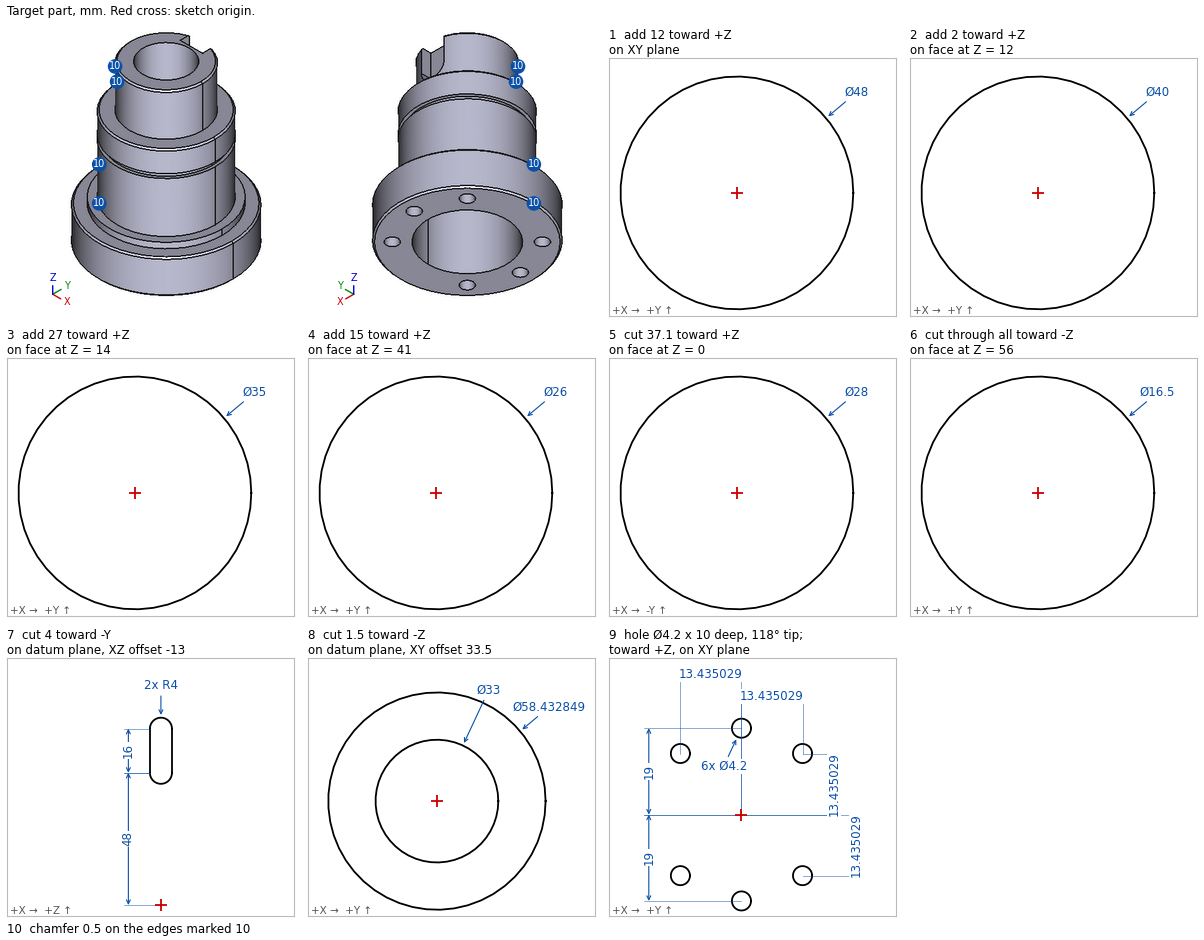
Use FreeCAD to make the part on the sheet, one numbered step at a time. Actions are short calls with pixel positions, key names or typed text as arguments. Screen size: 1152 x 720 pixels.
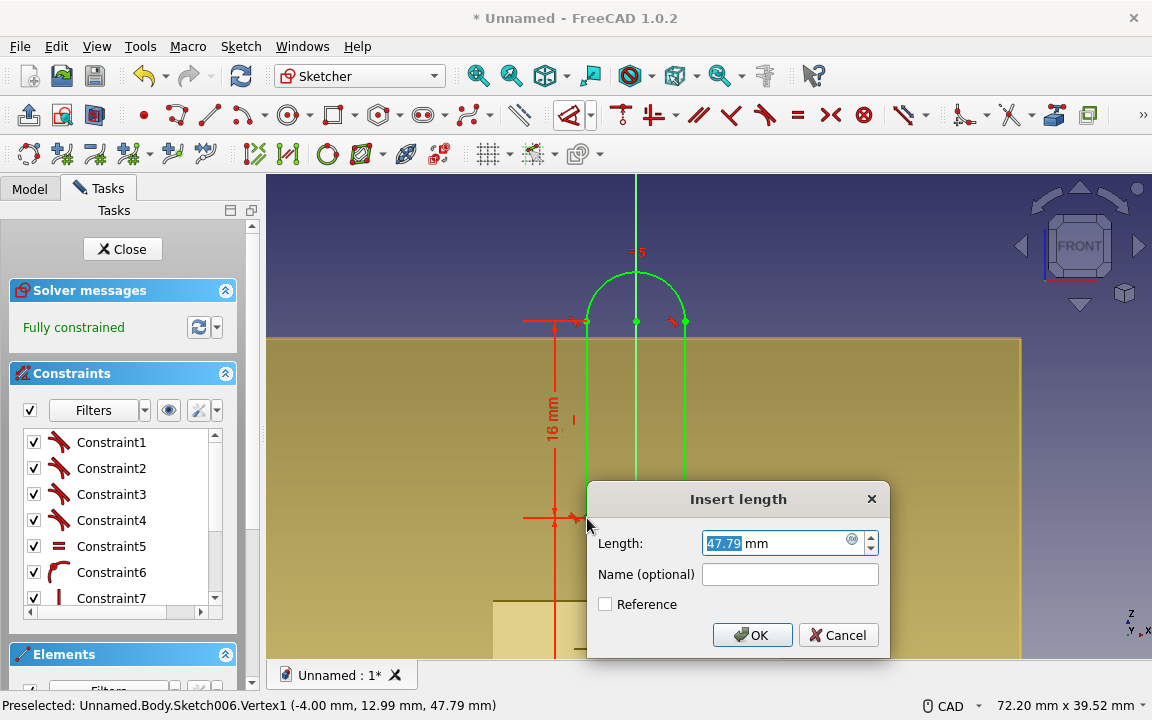
text(48)
key(Return)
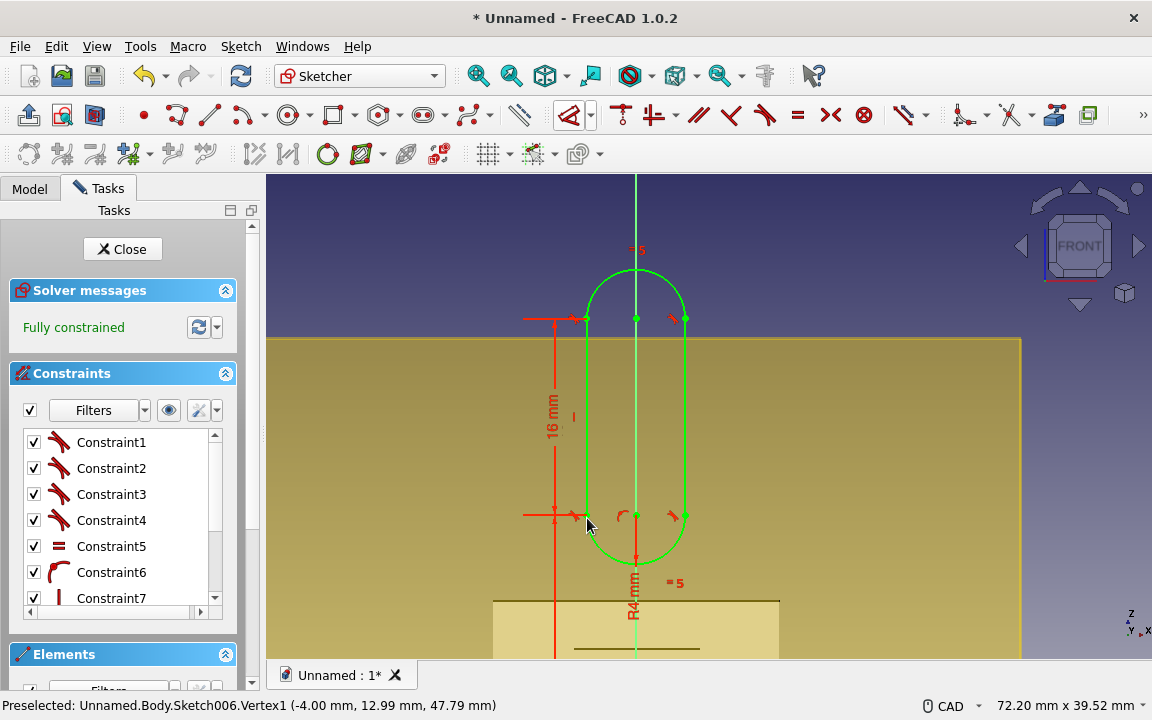
click(123, 249)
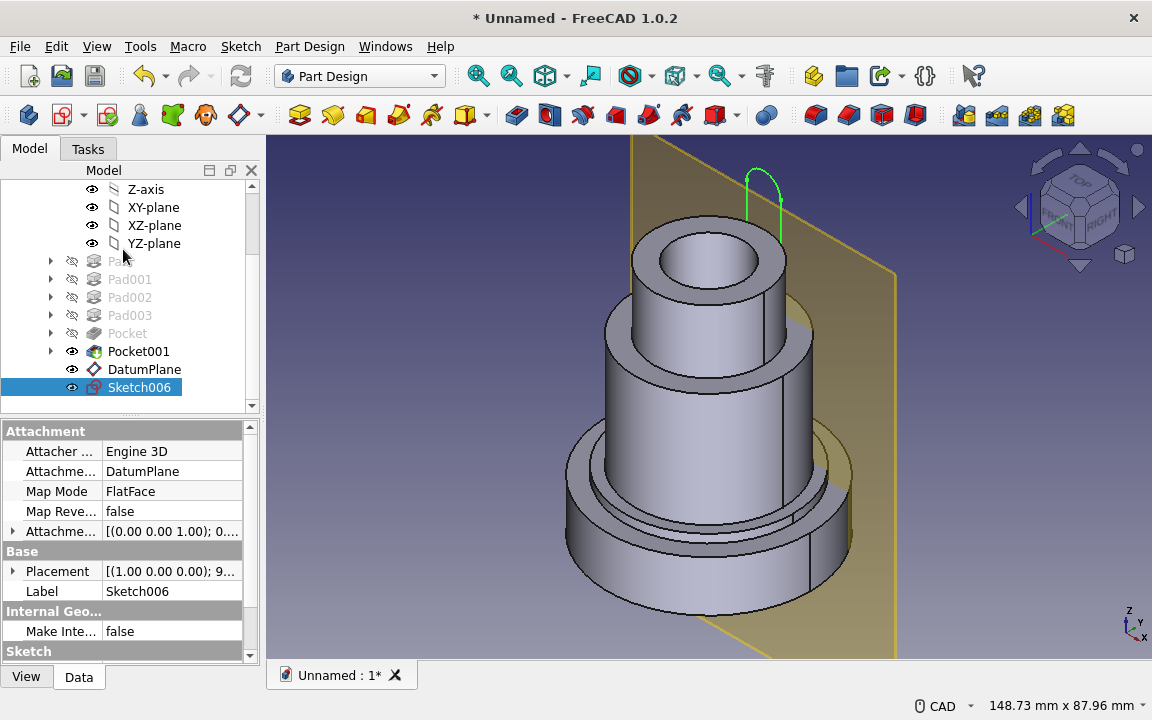
click(517, 116)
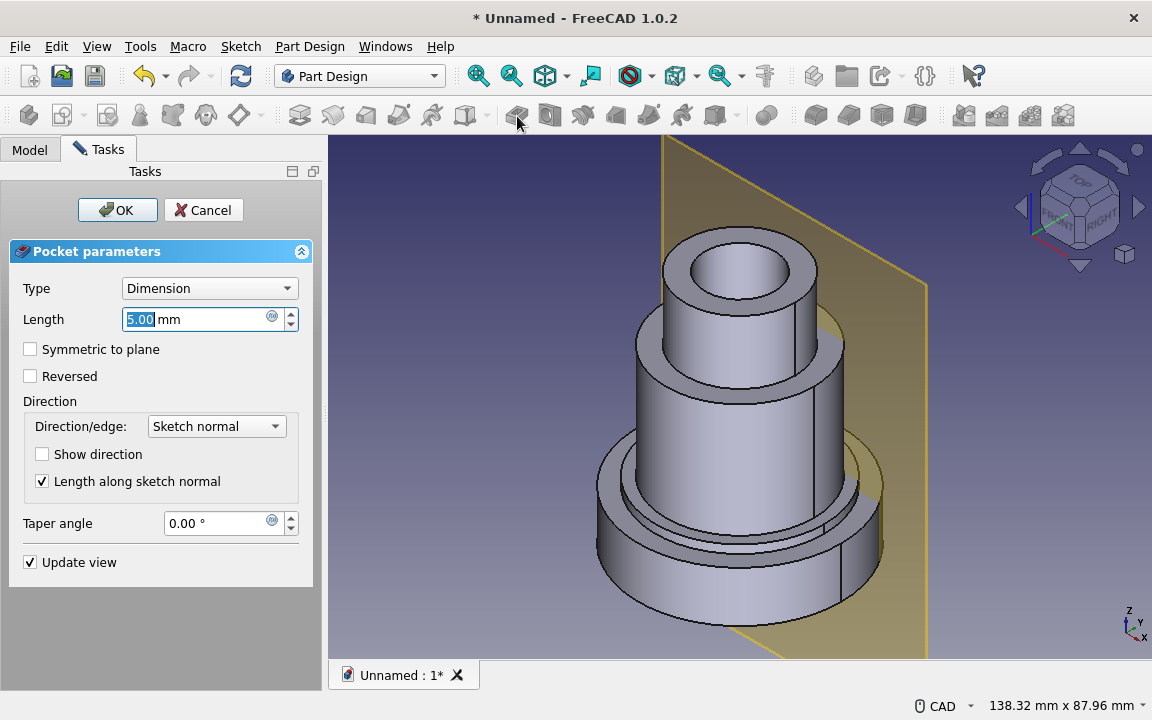
text(4)
key(Tab)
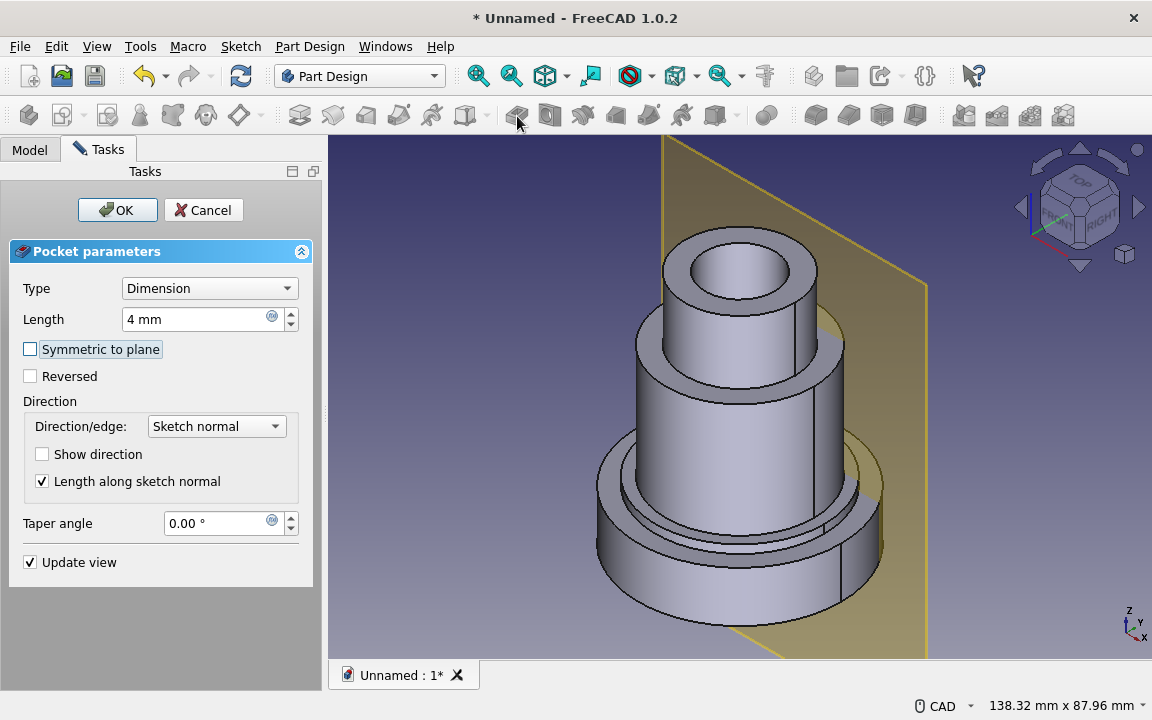
click(31, 376)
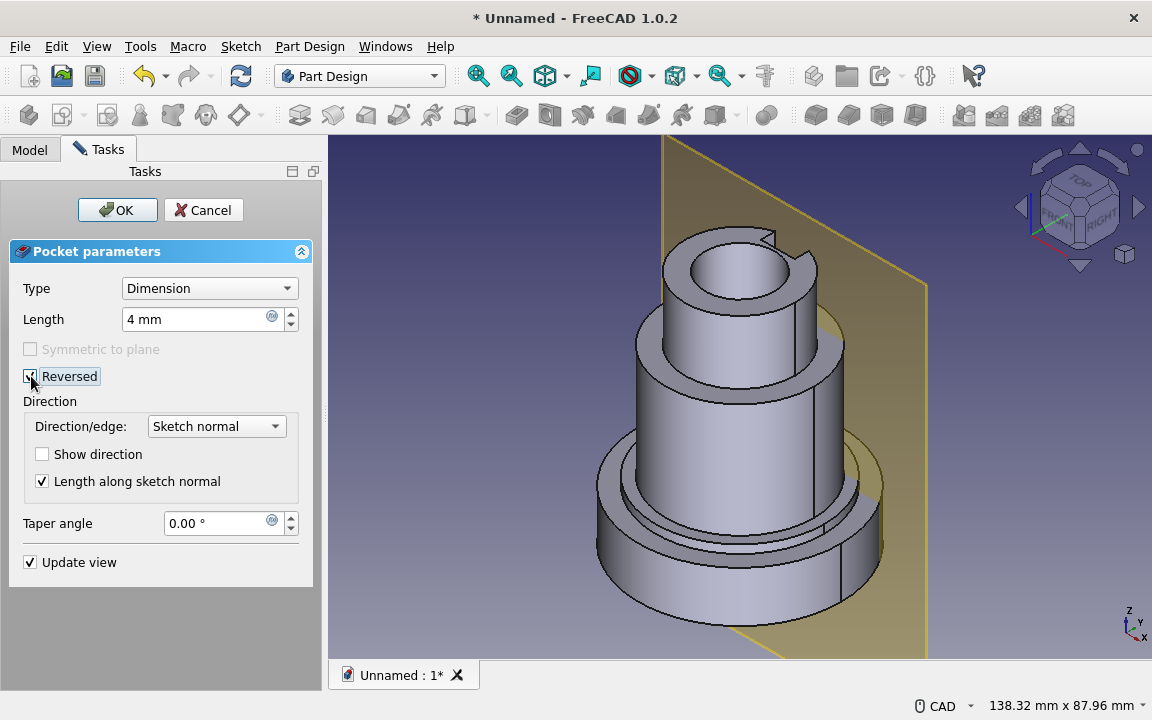
click(118, 210)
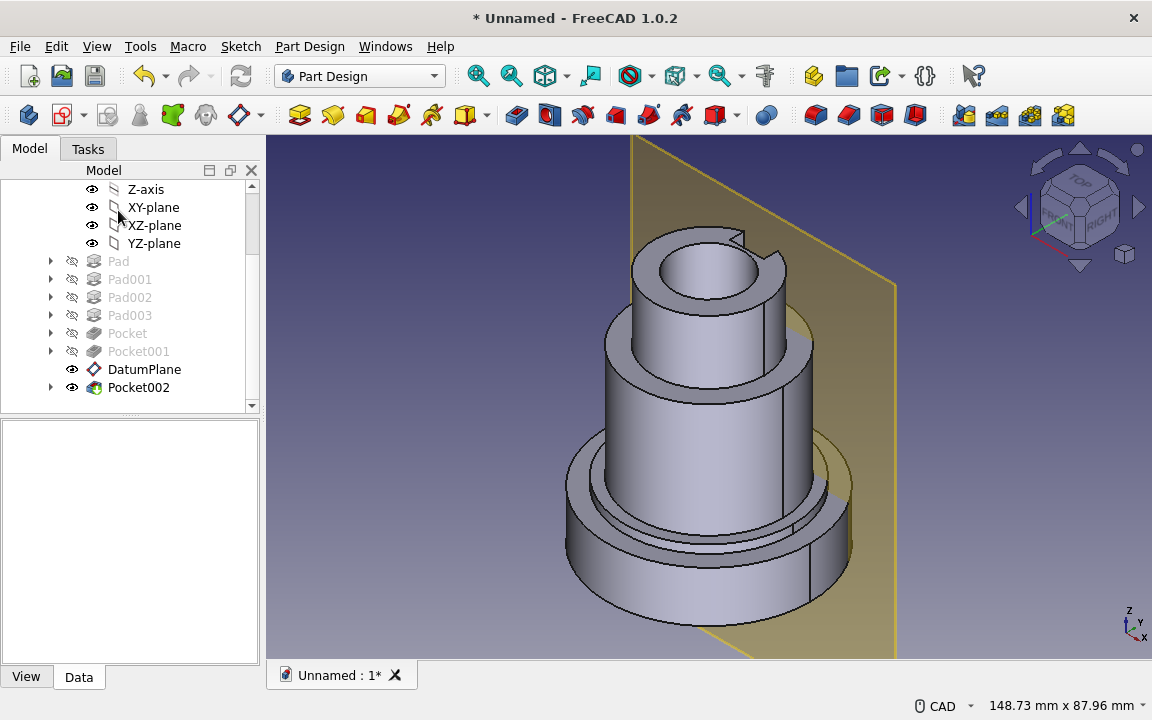
click(117, 369)
key(space)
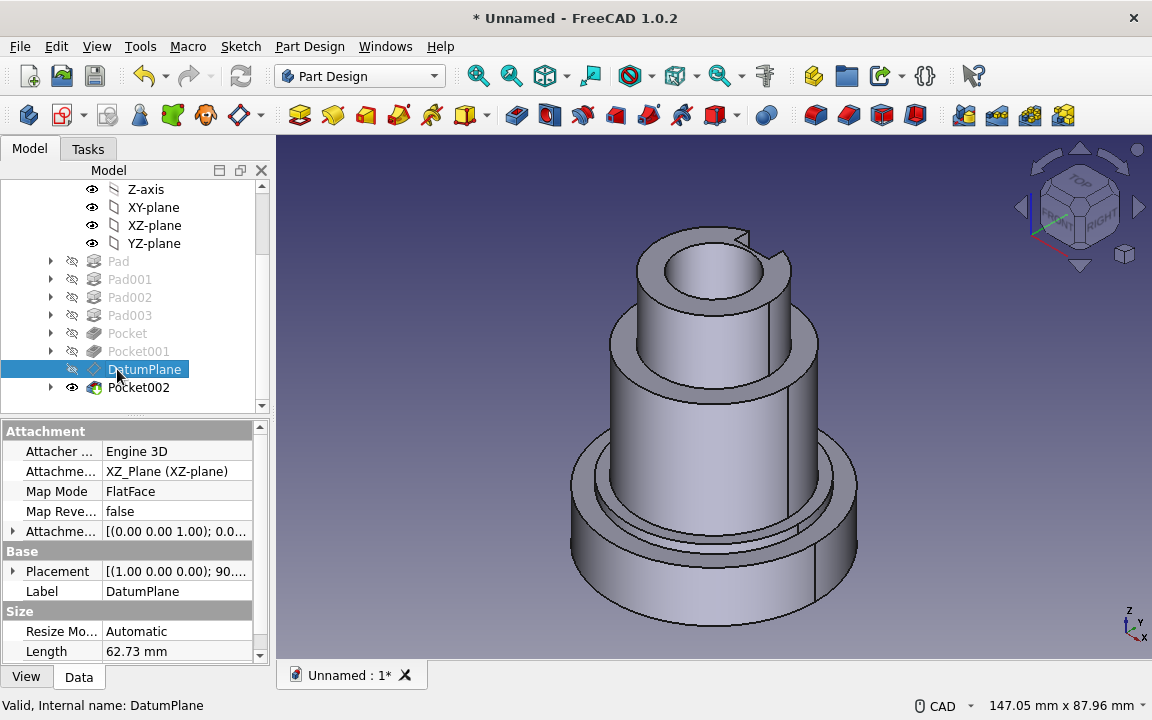
scroll(161, 293, down, 3)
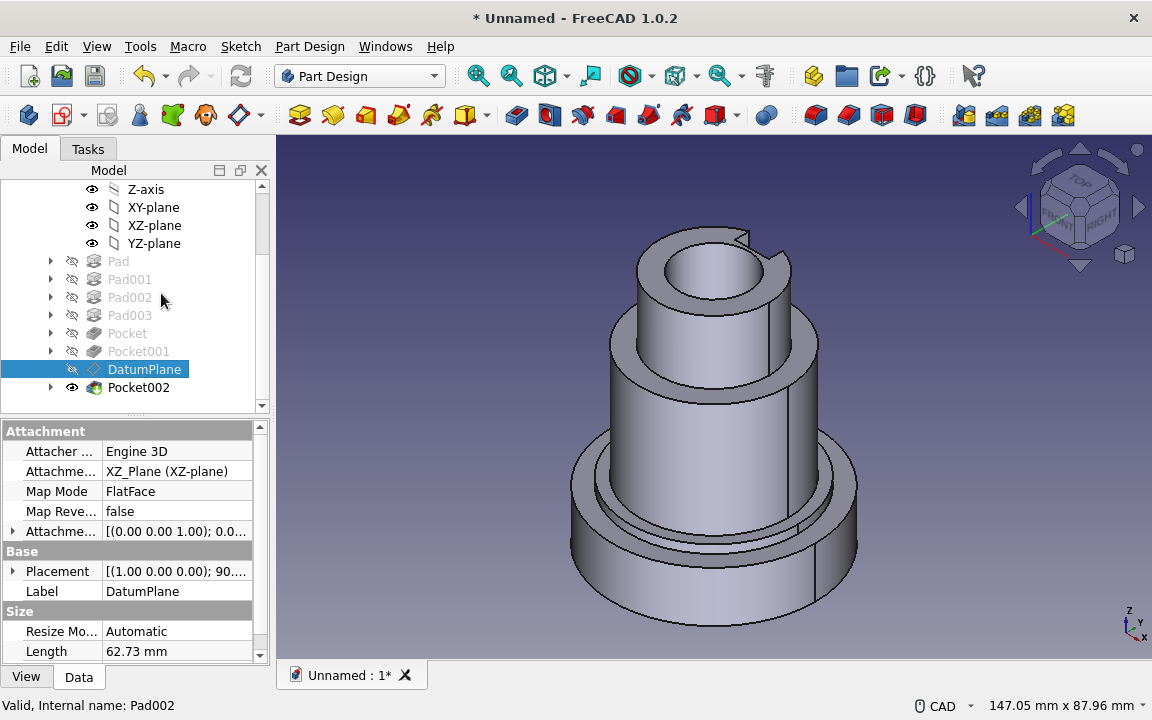
scroll(161, 293, up, 15)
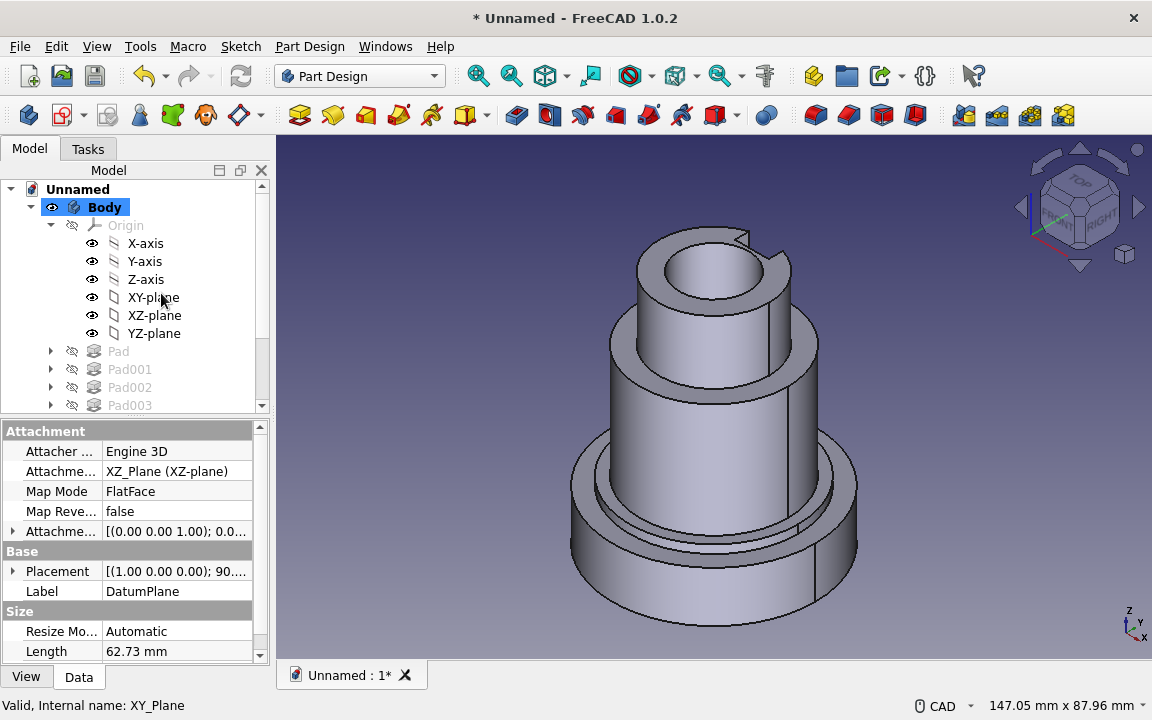
click(137, 297)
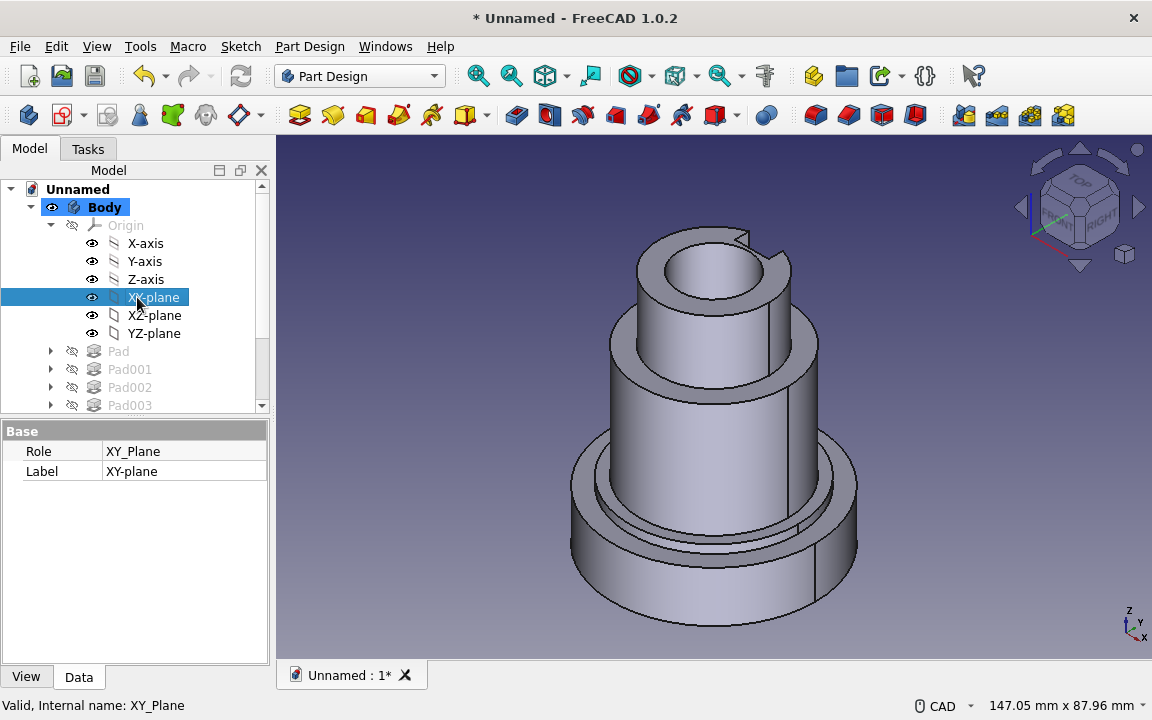
click(238, 116)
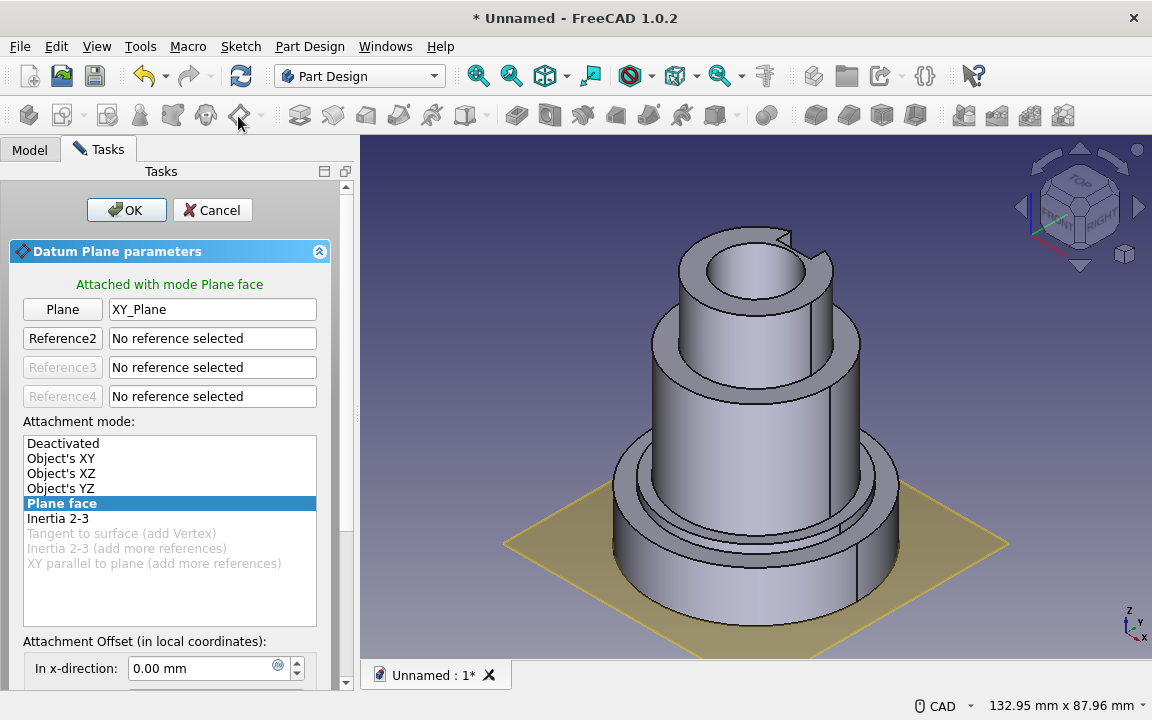
scroll(346, 436, down, 2)